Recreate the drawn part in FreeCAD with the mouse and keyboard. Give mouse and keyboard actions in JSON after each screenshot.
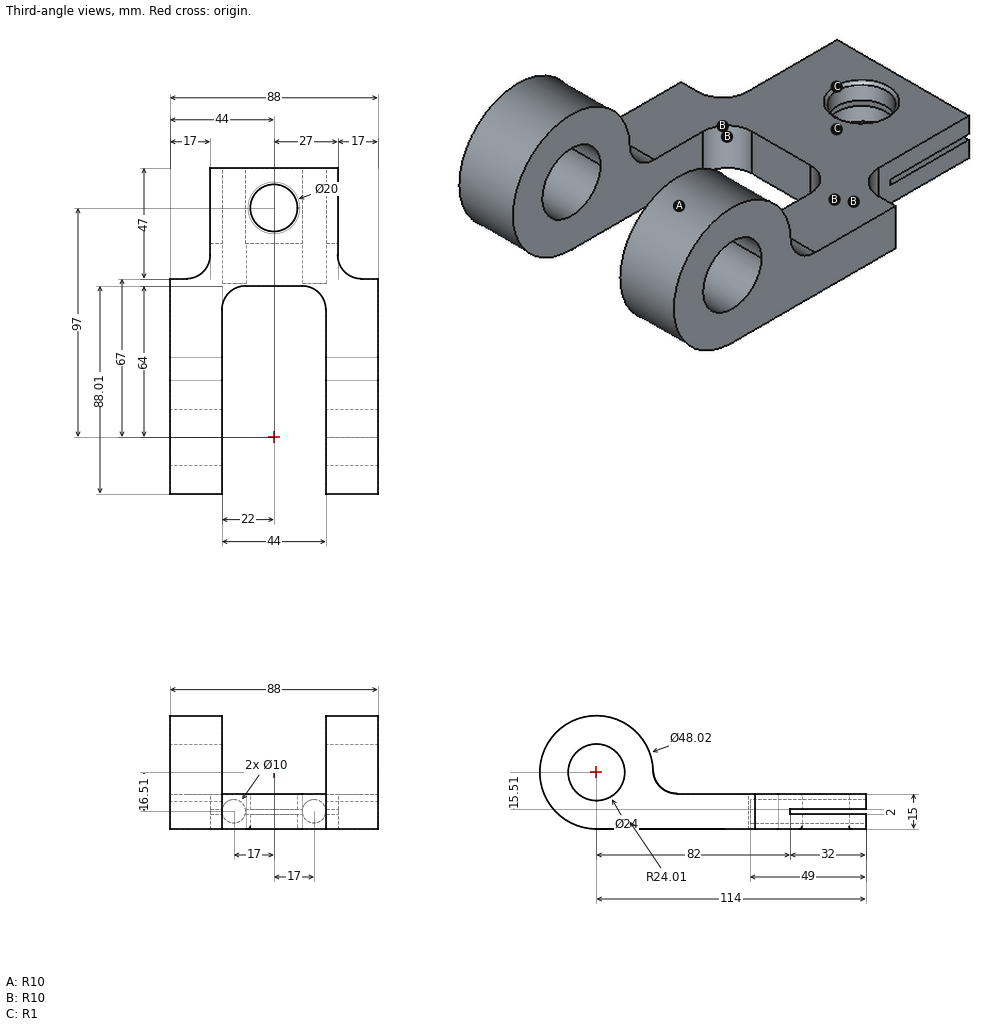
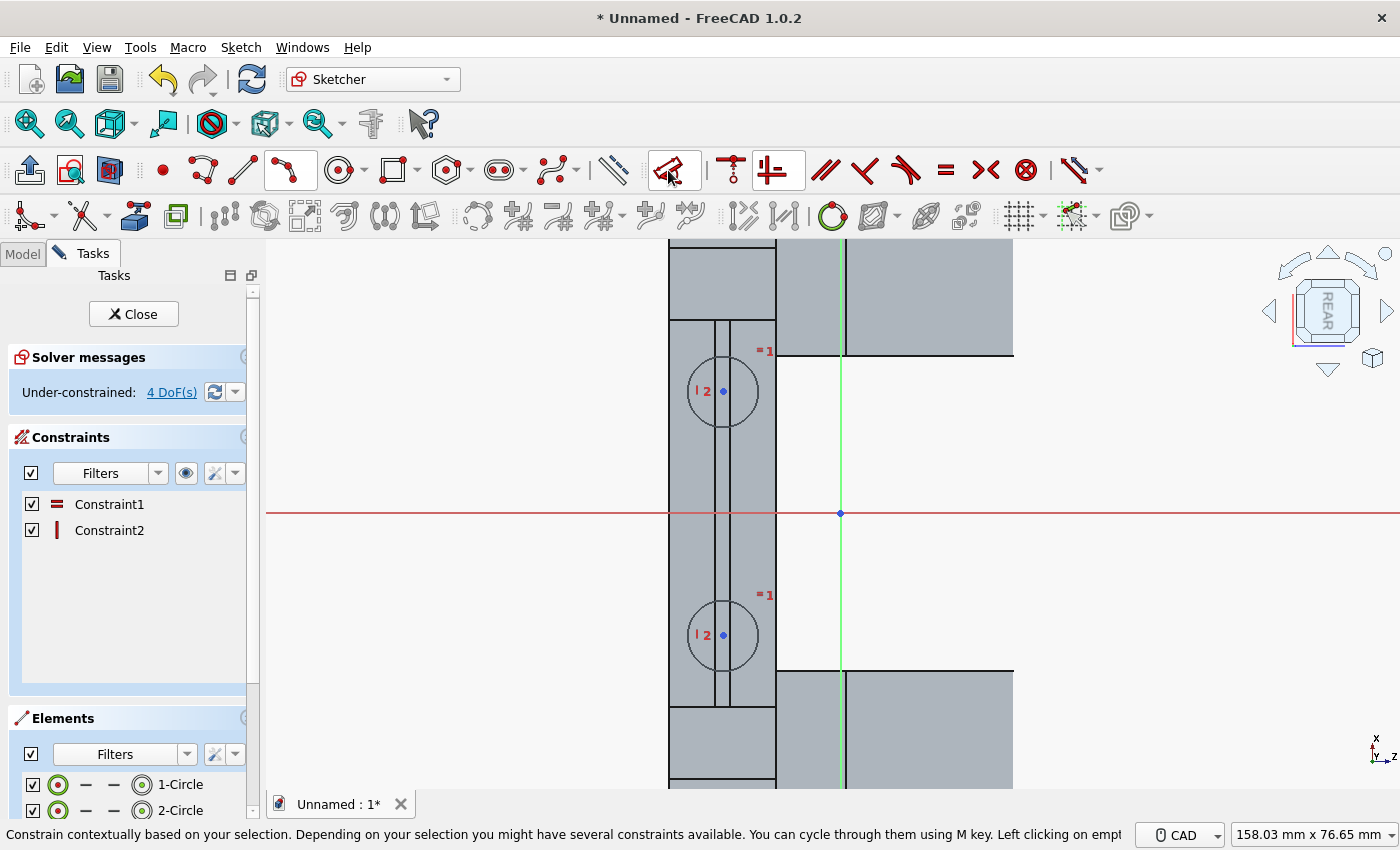
{"action": "left_click", "coordinate": [748, 611]}
{"action": "left_click", "coordinate": [771, 588]}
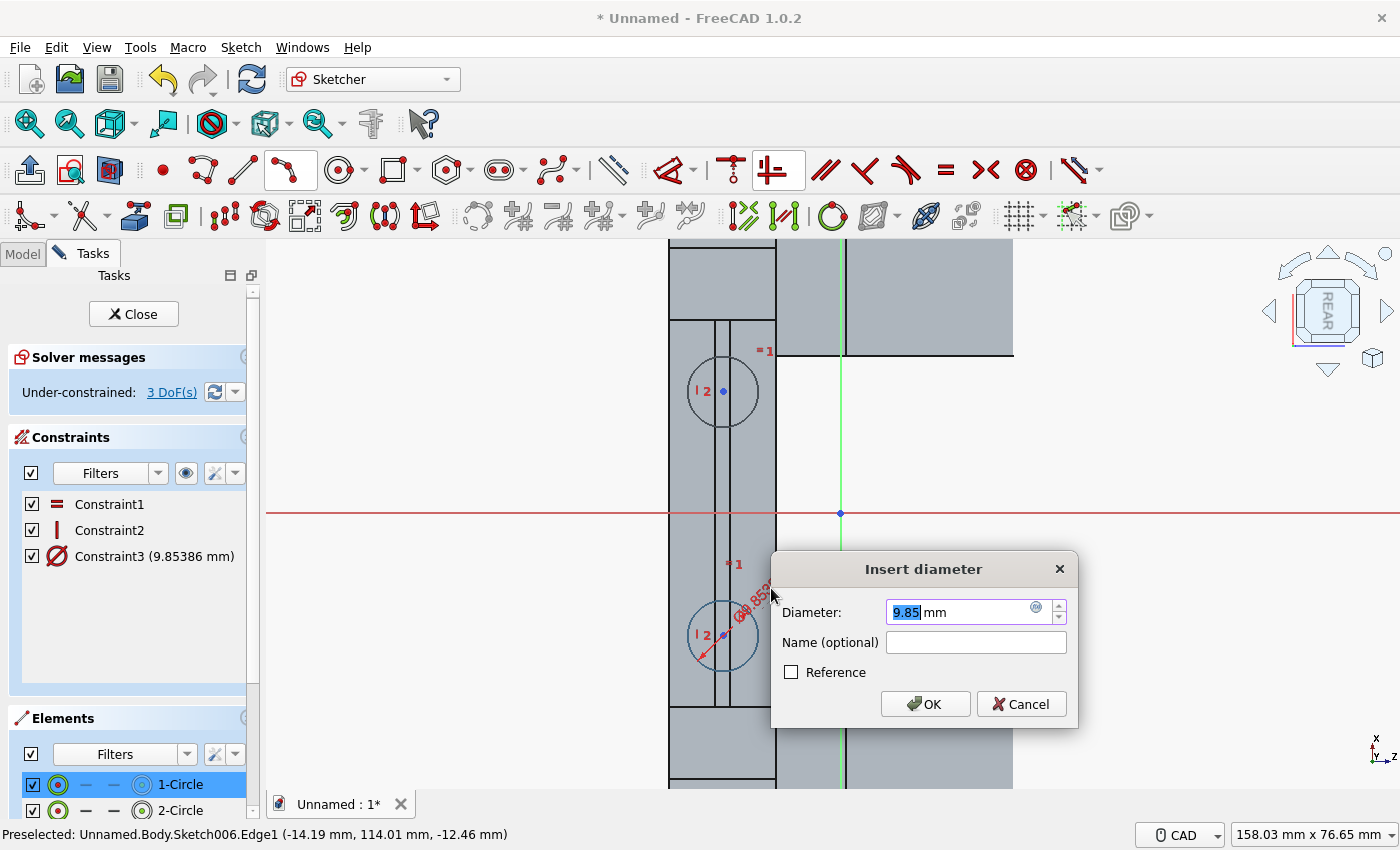
{"action": "type", "text": "10"}
{"action": "key", "text": "Return"}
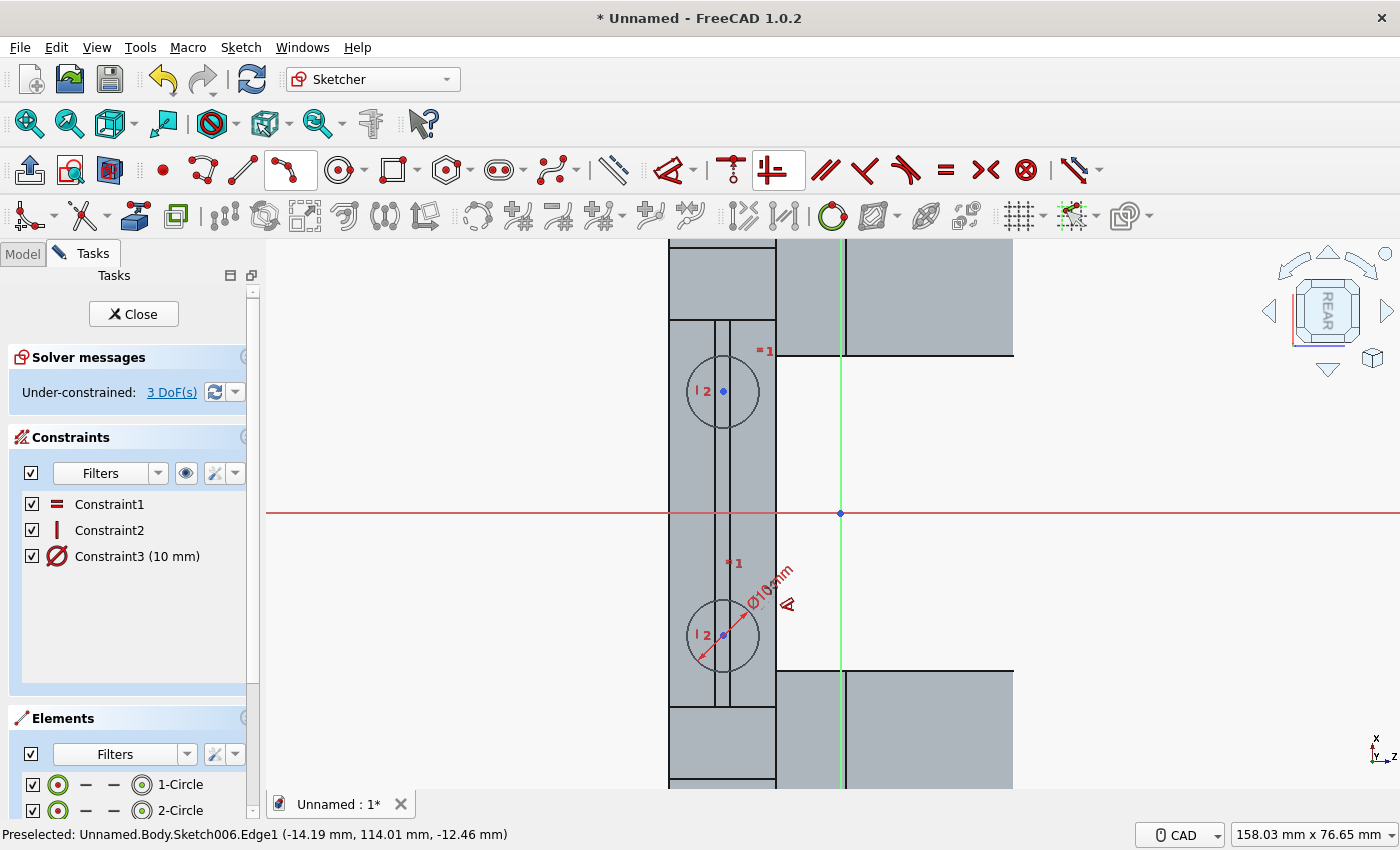
{"action": "left_click", "coordinate": [723, 636]}
{"action": "left_click", "coordinate": [875, 575]}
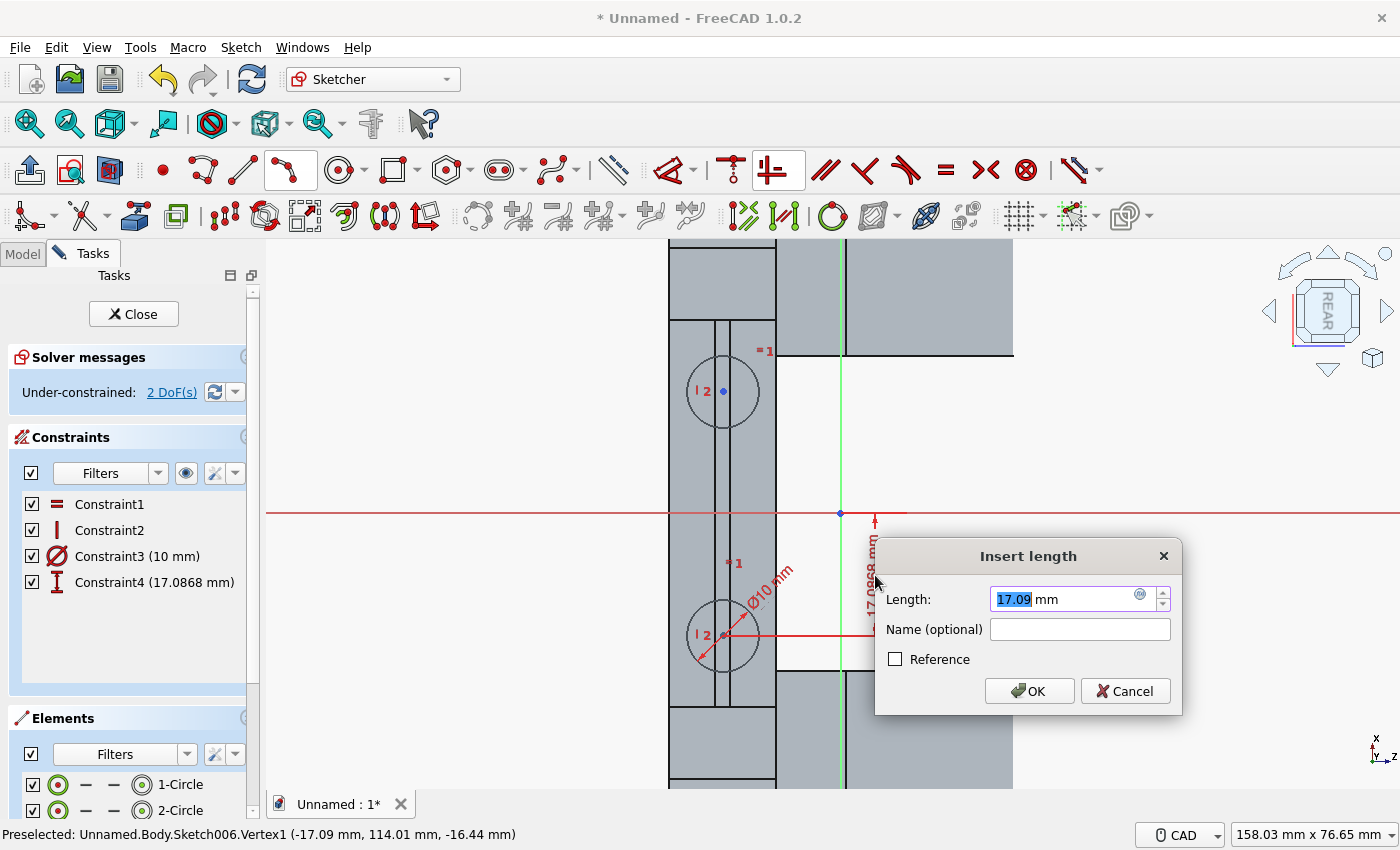
{"action": "type", "text": "17"}
{"action": "key", "text": "Return"}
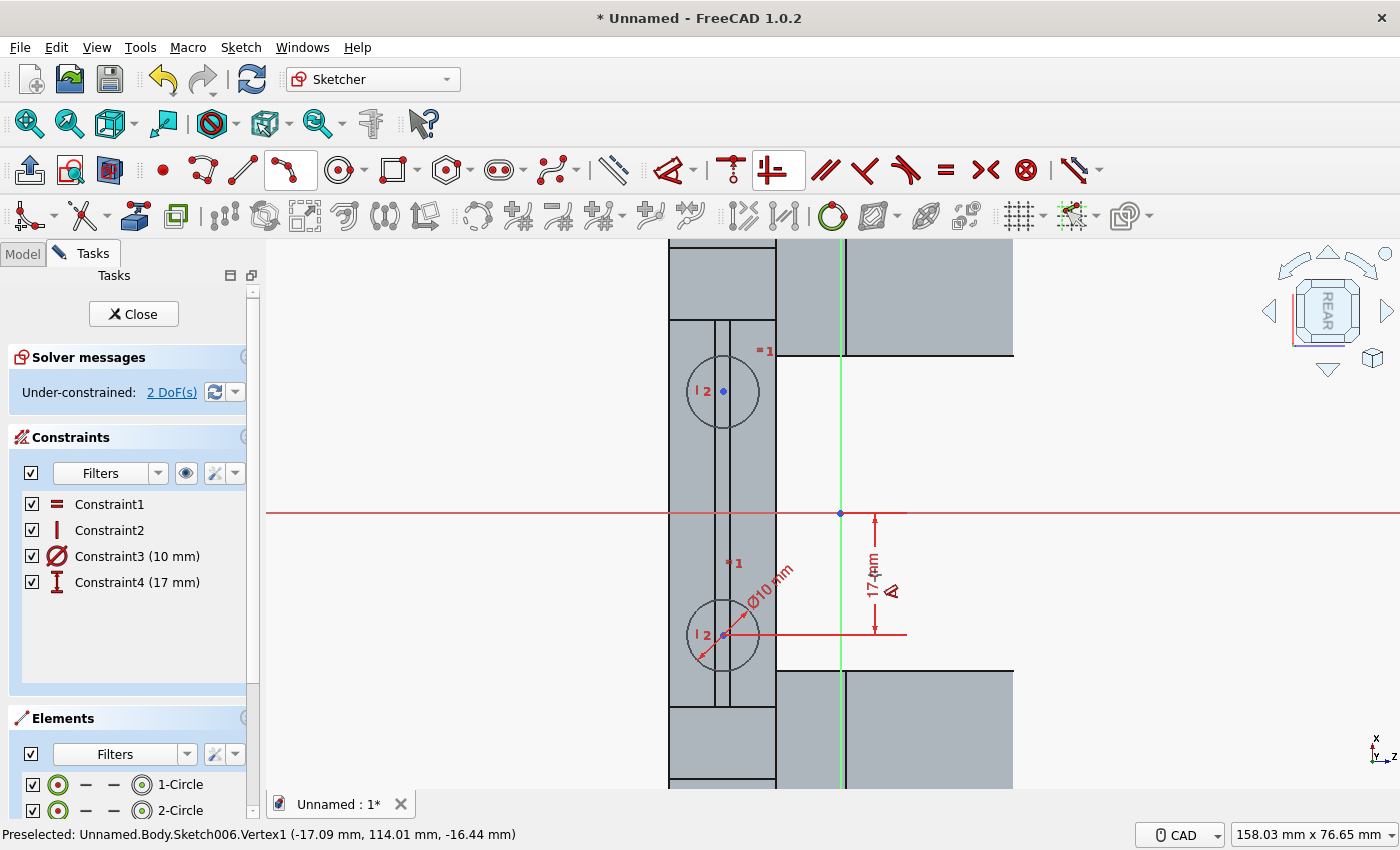
{"action": "left_click", "coordinate": [723, 392]}
{"action": "left_click", "coordinate": [875, 453]}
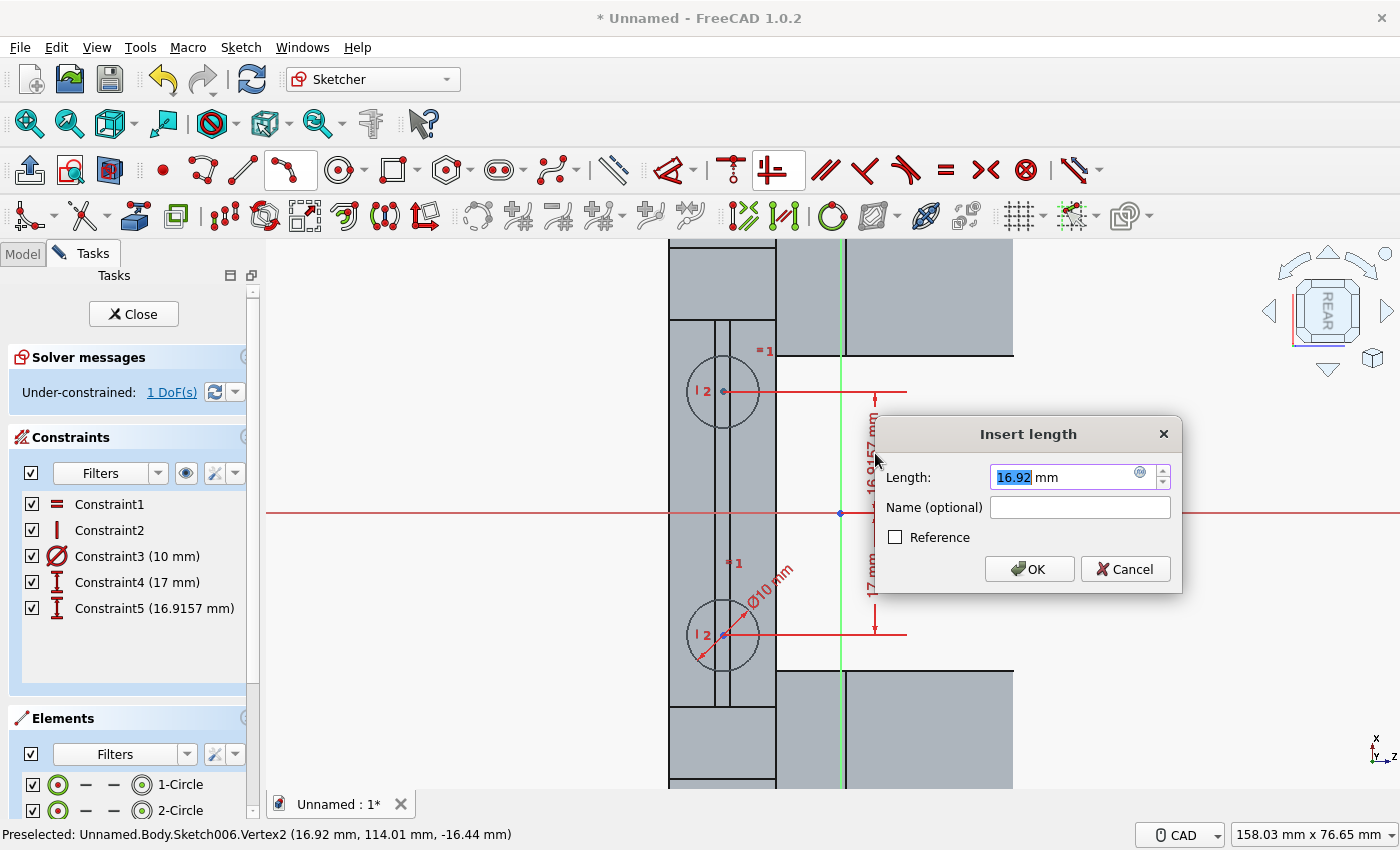
{"action": "type", "text": "17"}
{"action": "key", "text": "Return"}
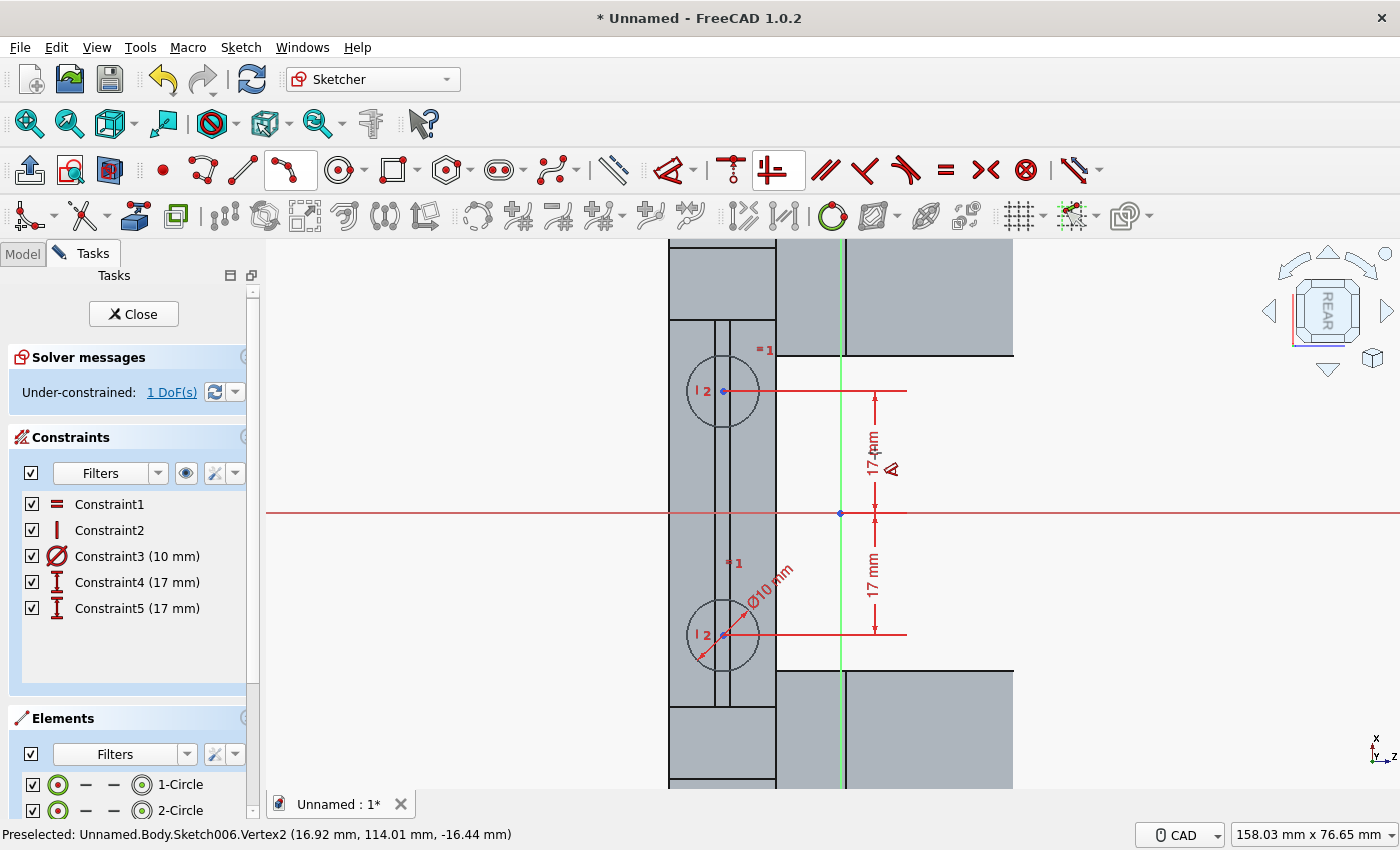
{"action": "left_click", "coordinate": [723, 635]}
{"action": "left_click", "coordinate": [782, 669]}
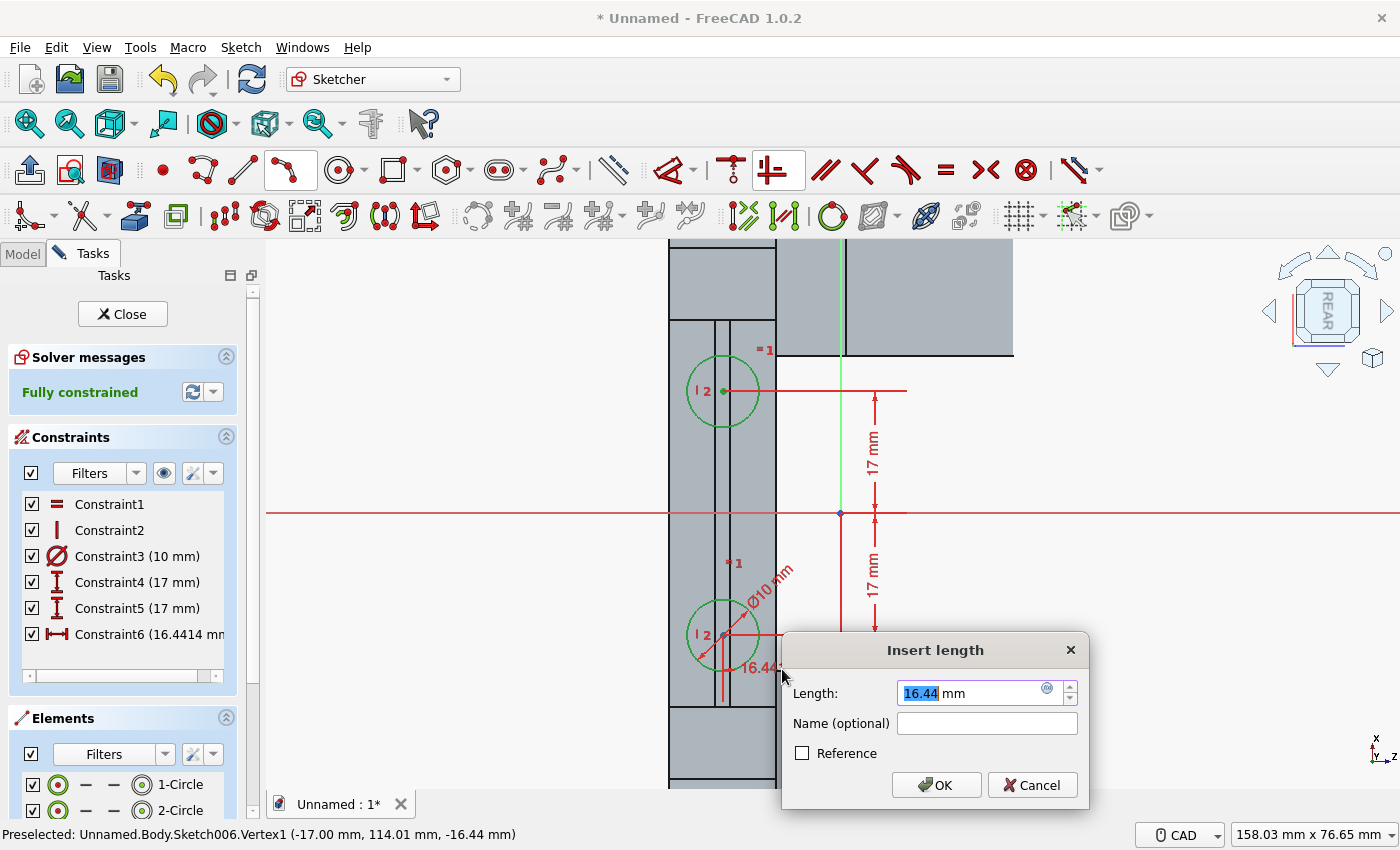
{"action": "type", "text": "16.51"}
{"action": "key", "text": "Return"}
{"action": "key", "text": "Escape"}